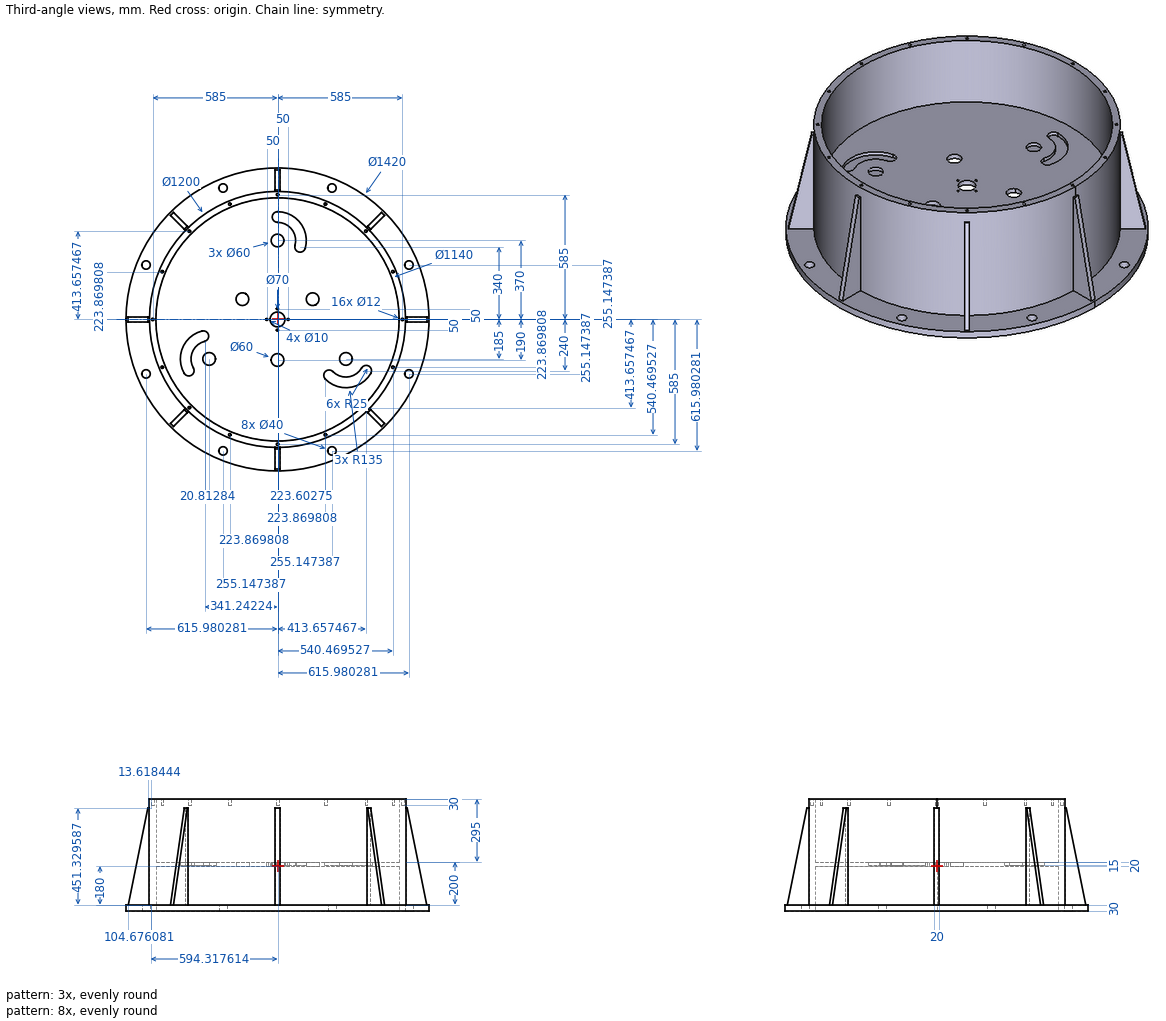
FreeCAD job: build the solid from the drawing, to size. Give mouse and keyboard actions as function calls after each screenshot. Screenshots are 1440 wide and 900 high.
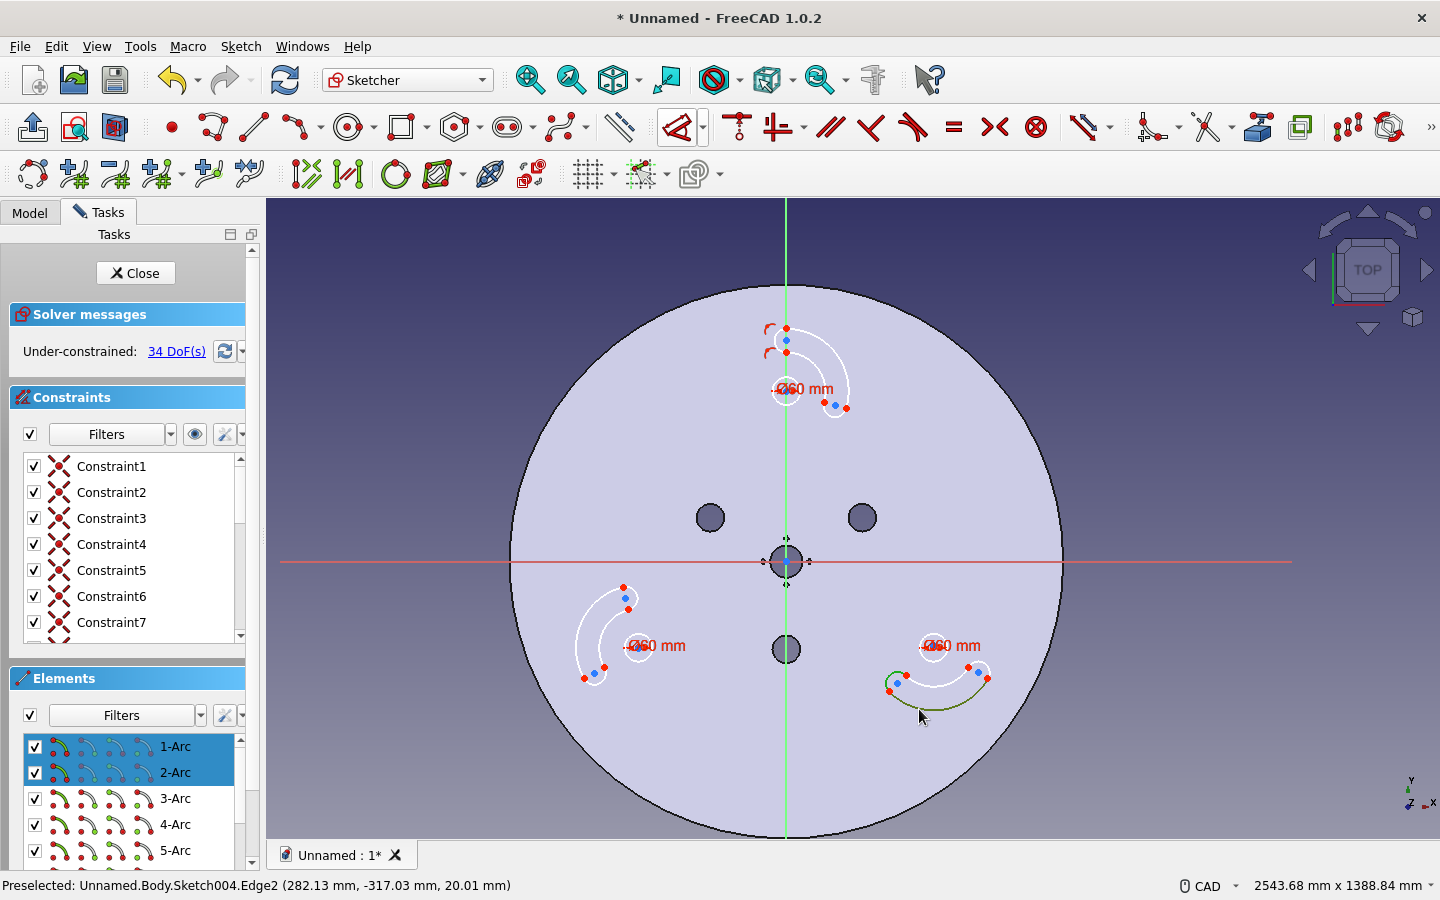
key(t)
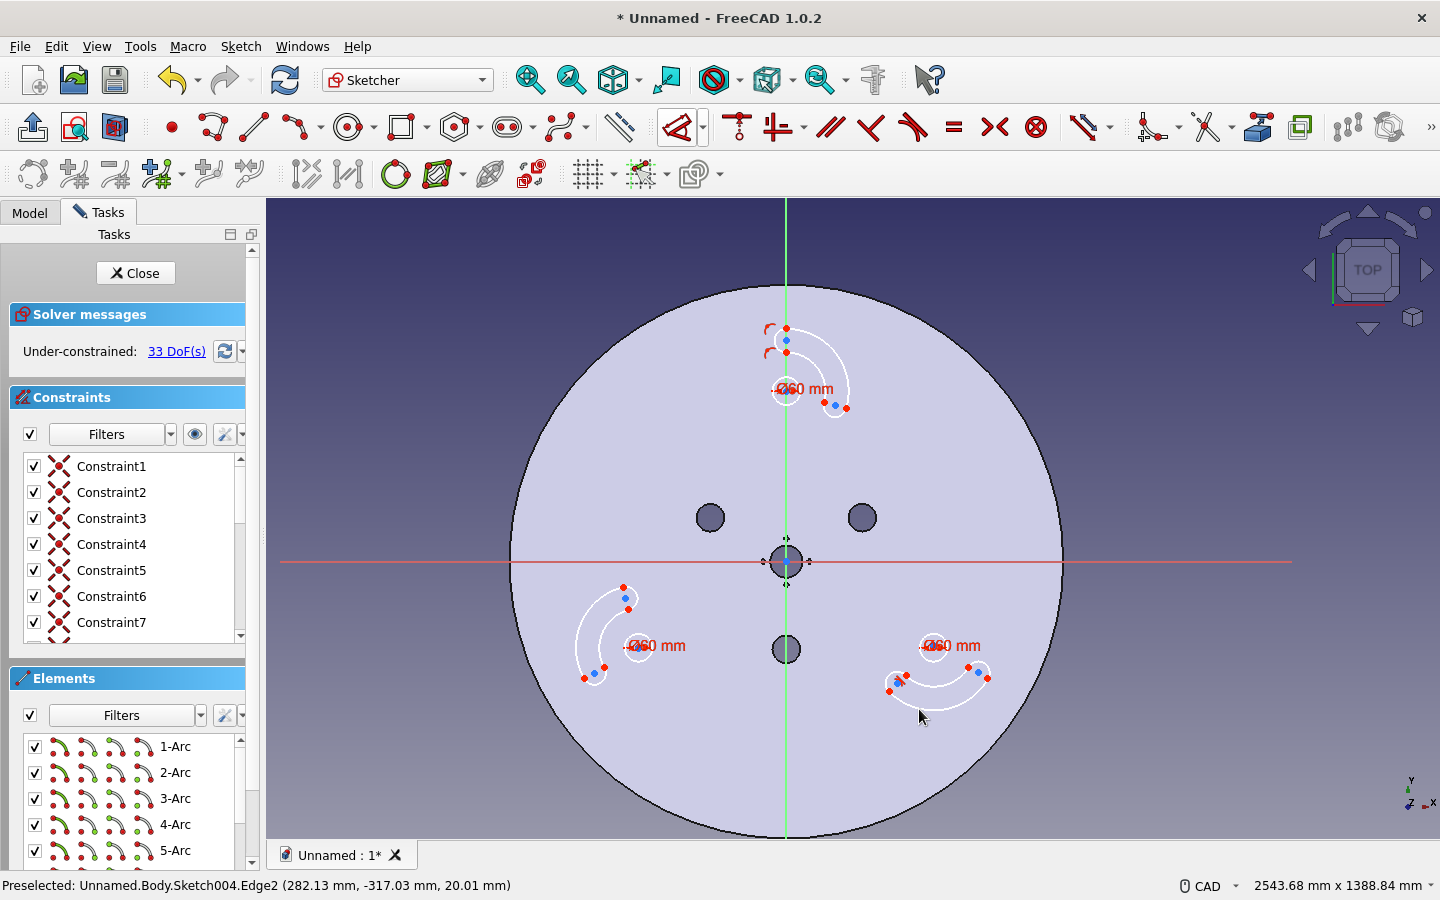
scroll(896, 672, up, 2)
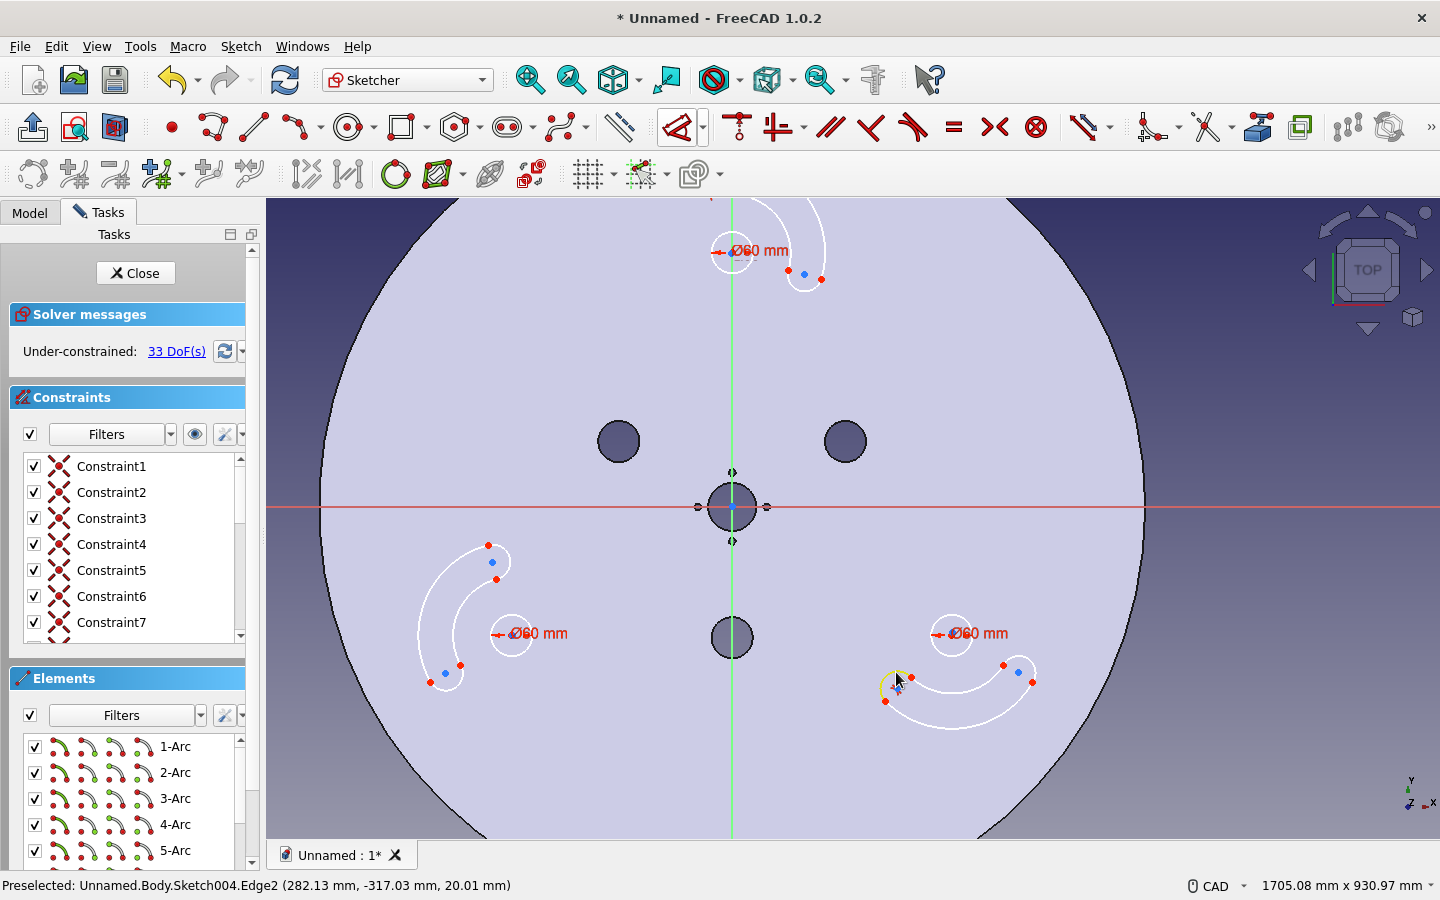
click(896, 671)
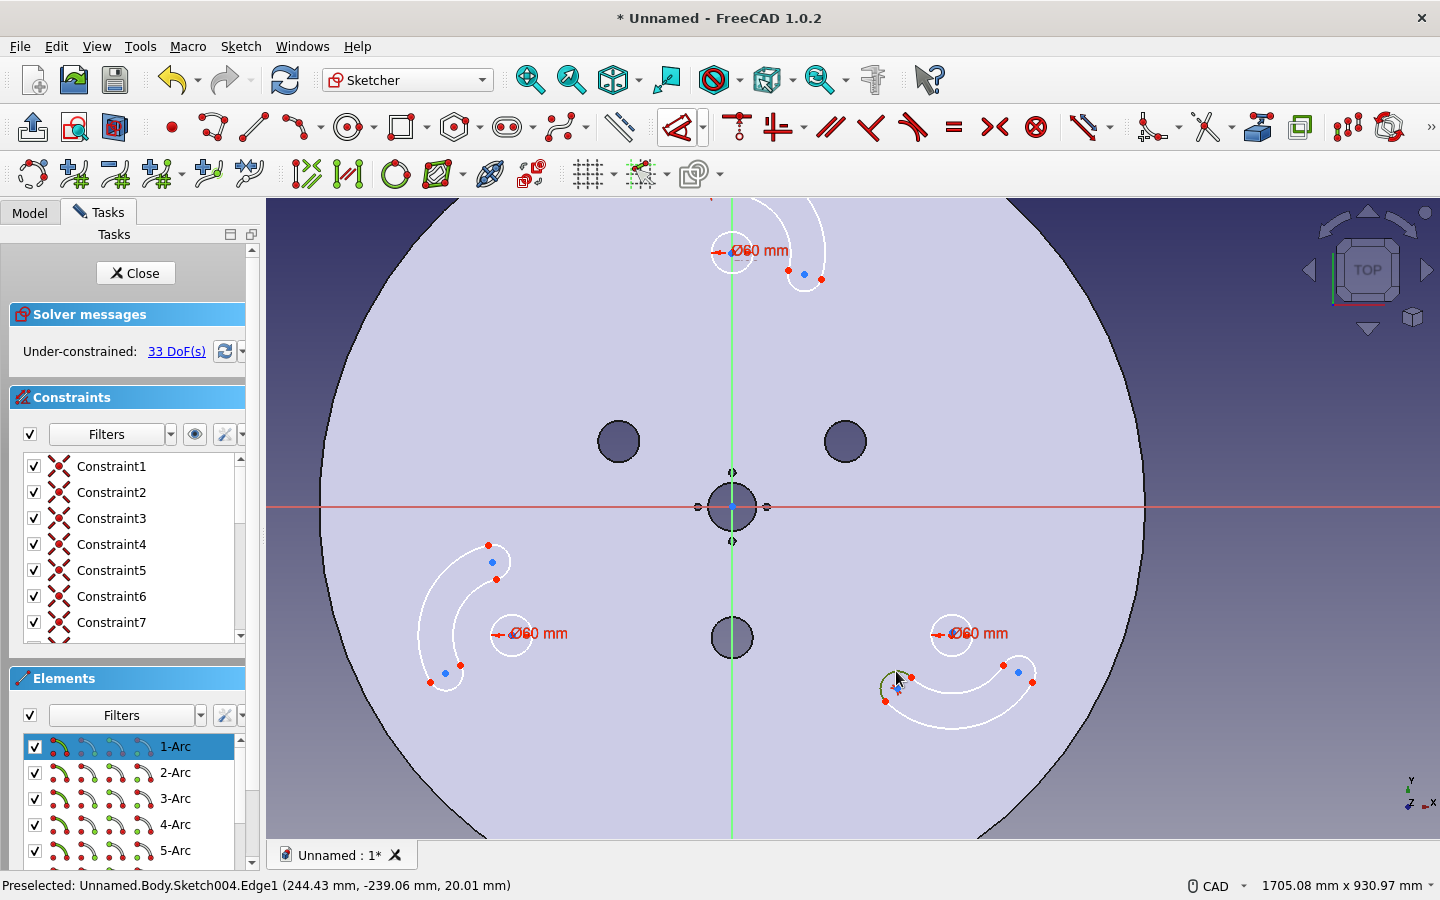
click(939, 692)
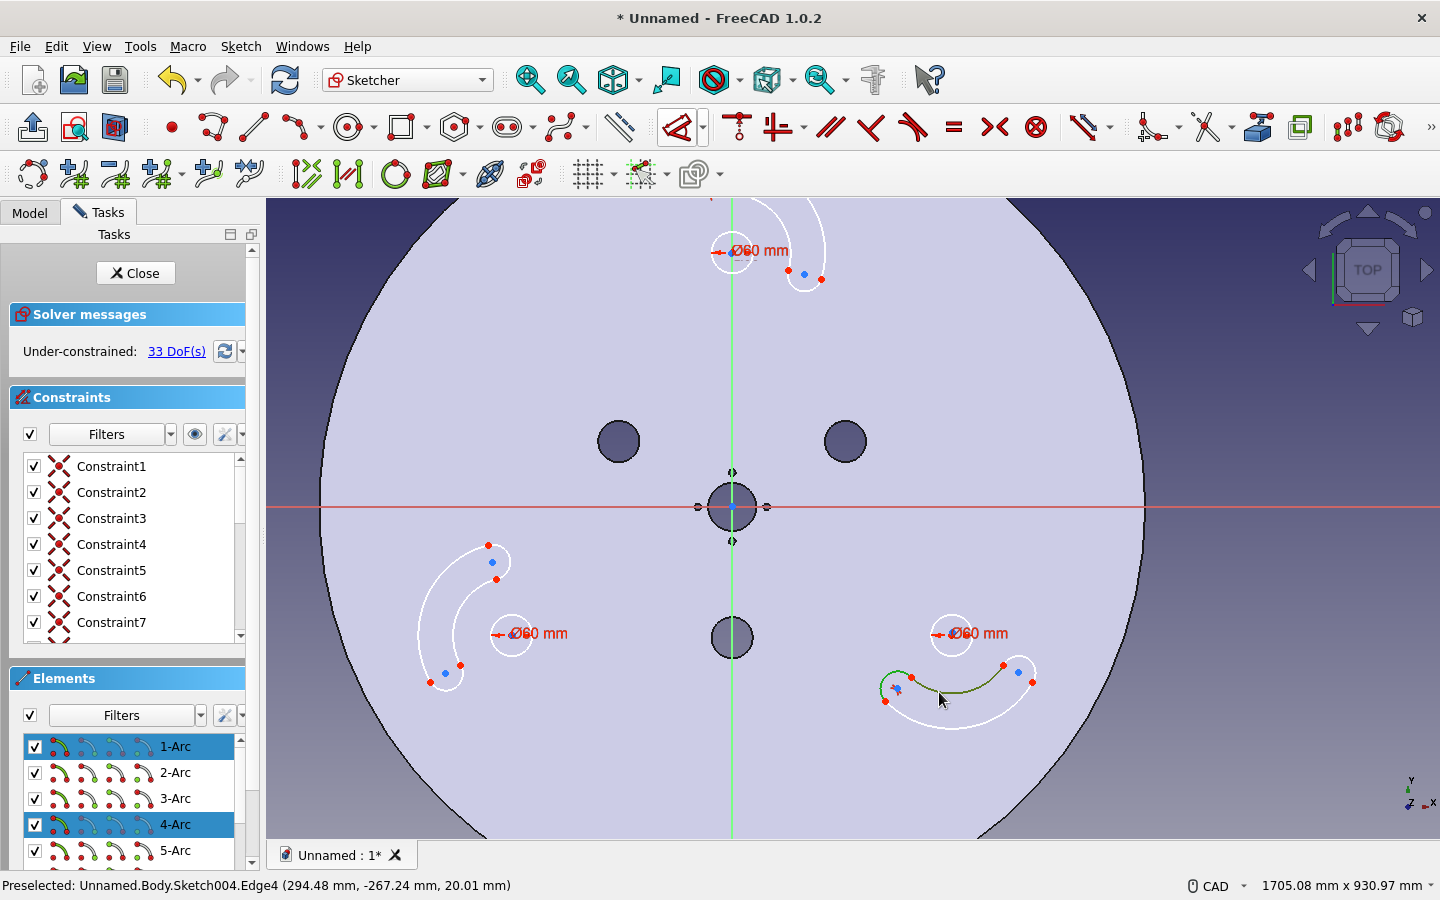
key(t)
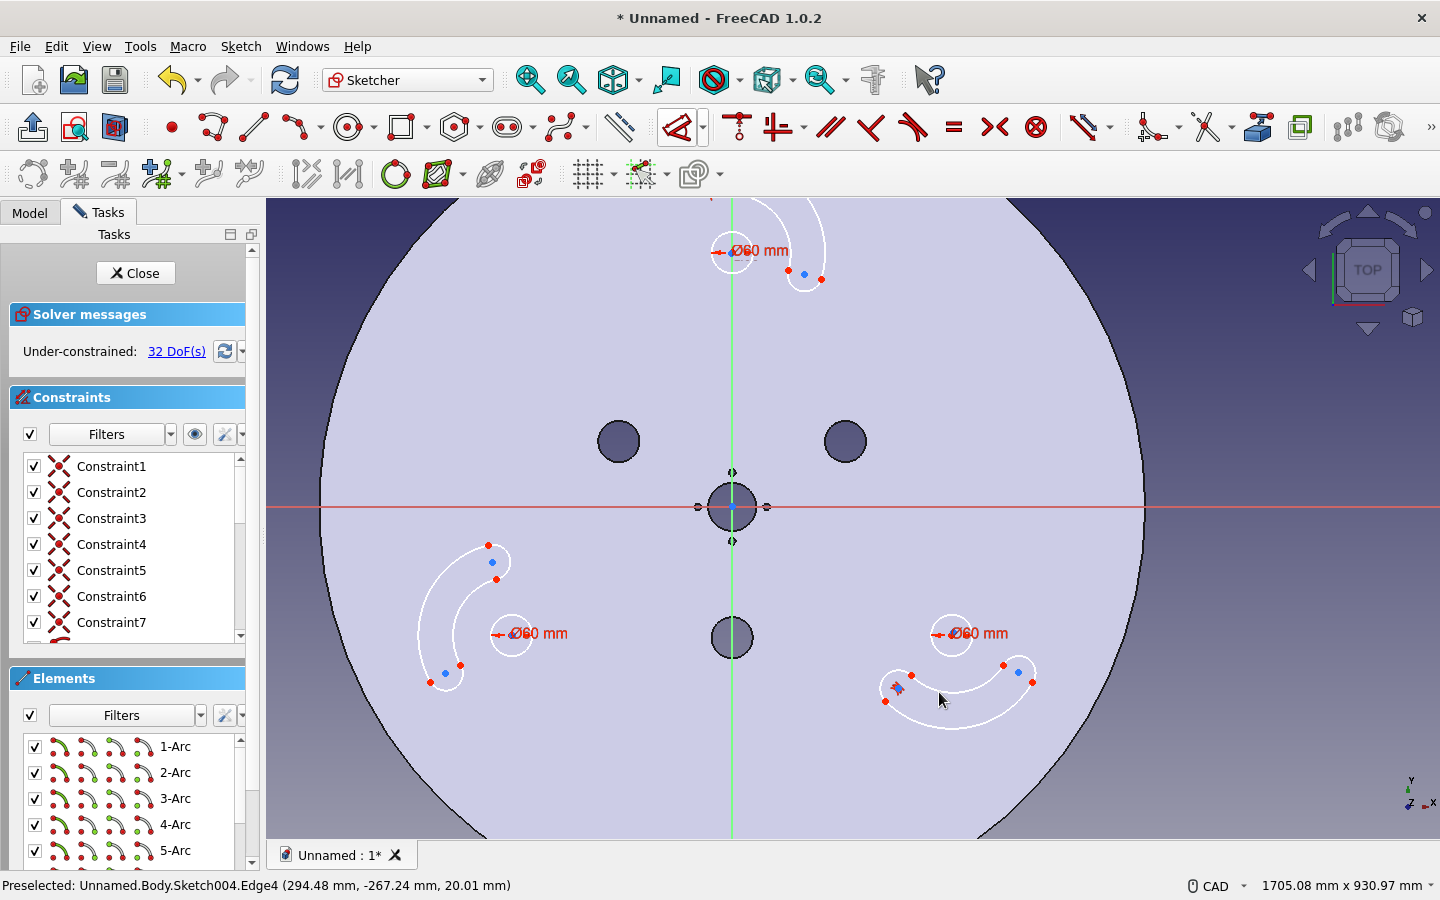
click(930, 726)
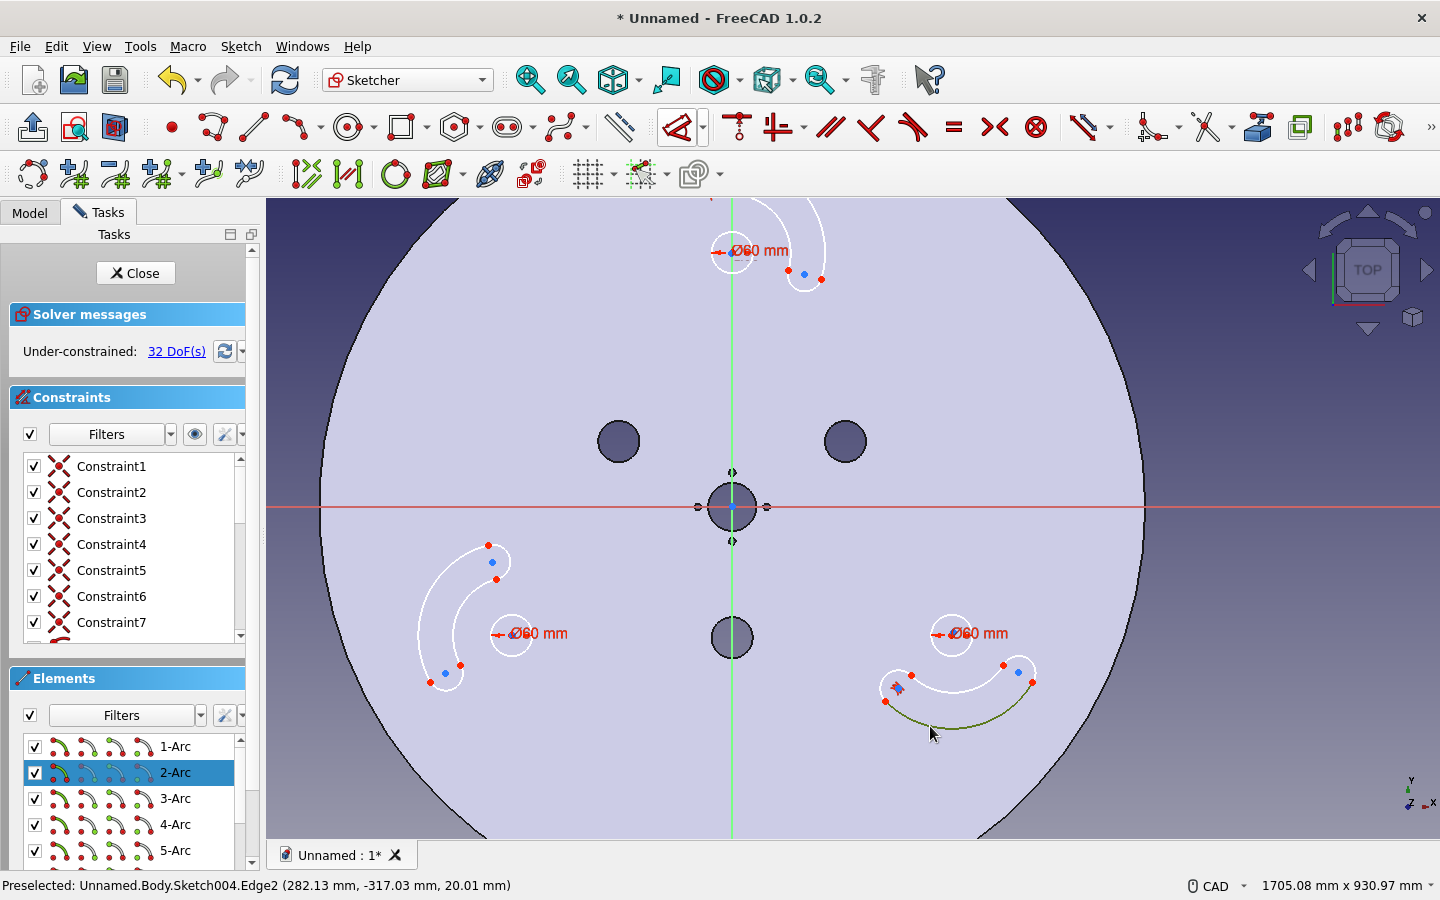
click(1034, 666)